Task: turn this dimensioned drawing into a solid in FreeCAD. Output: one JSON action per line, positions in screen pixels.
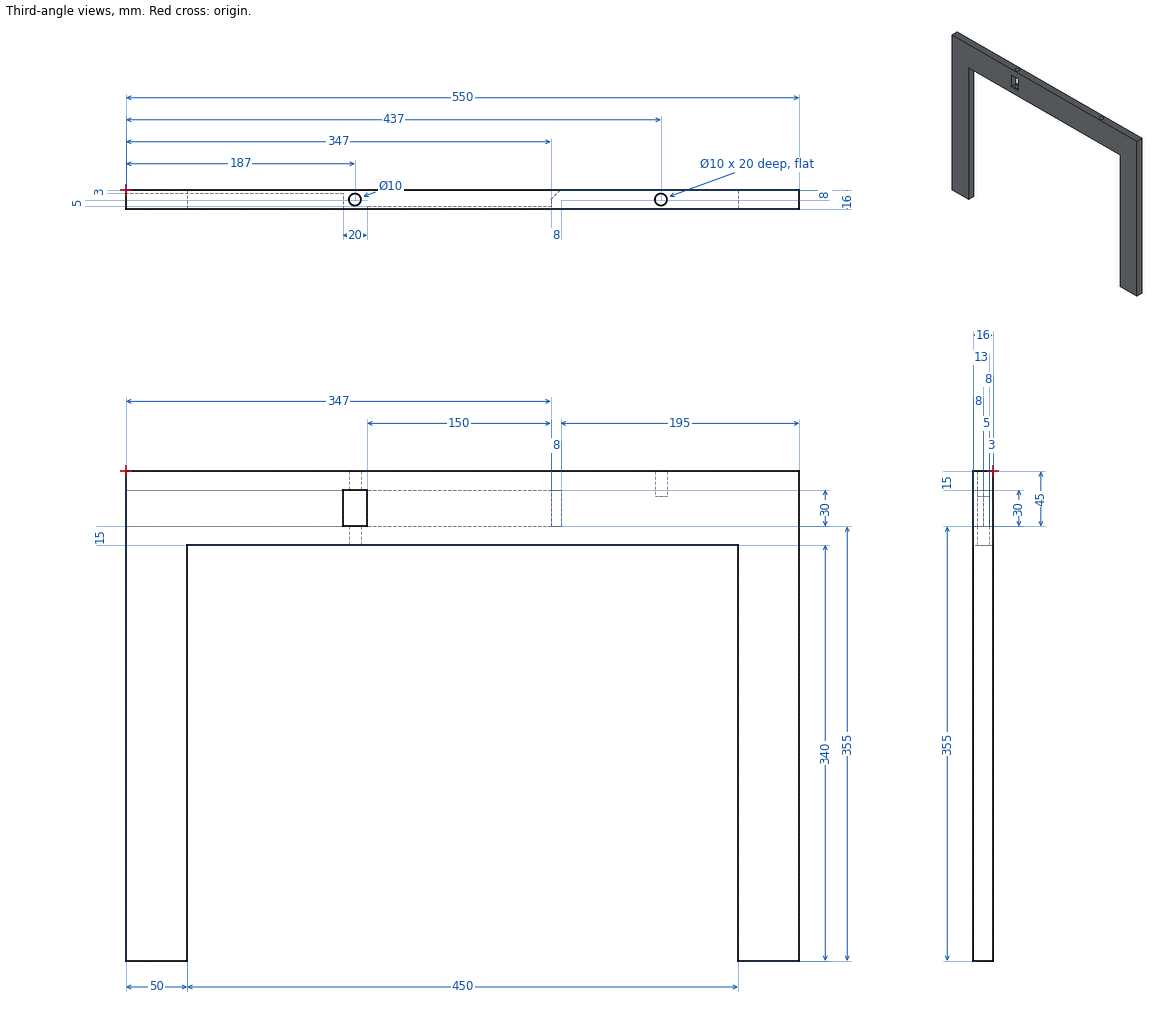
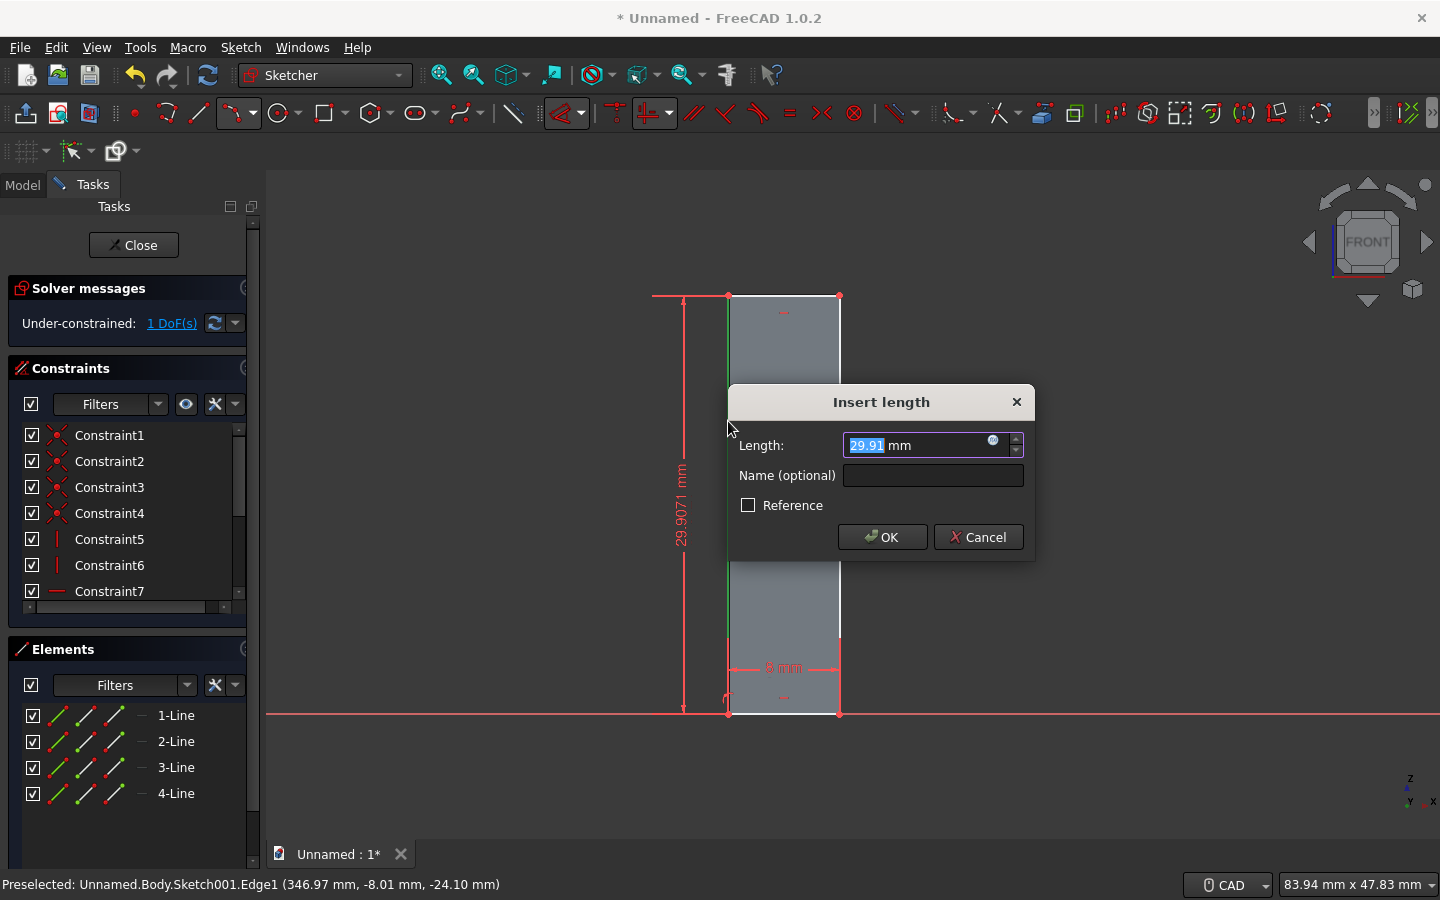
{"action": "type", "text": "30"}
{"action": "key", "text": "Return"}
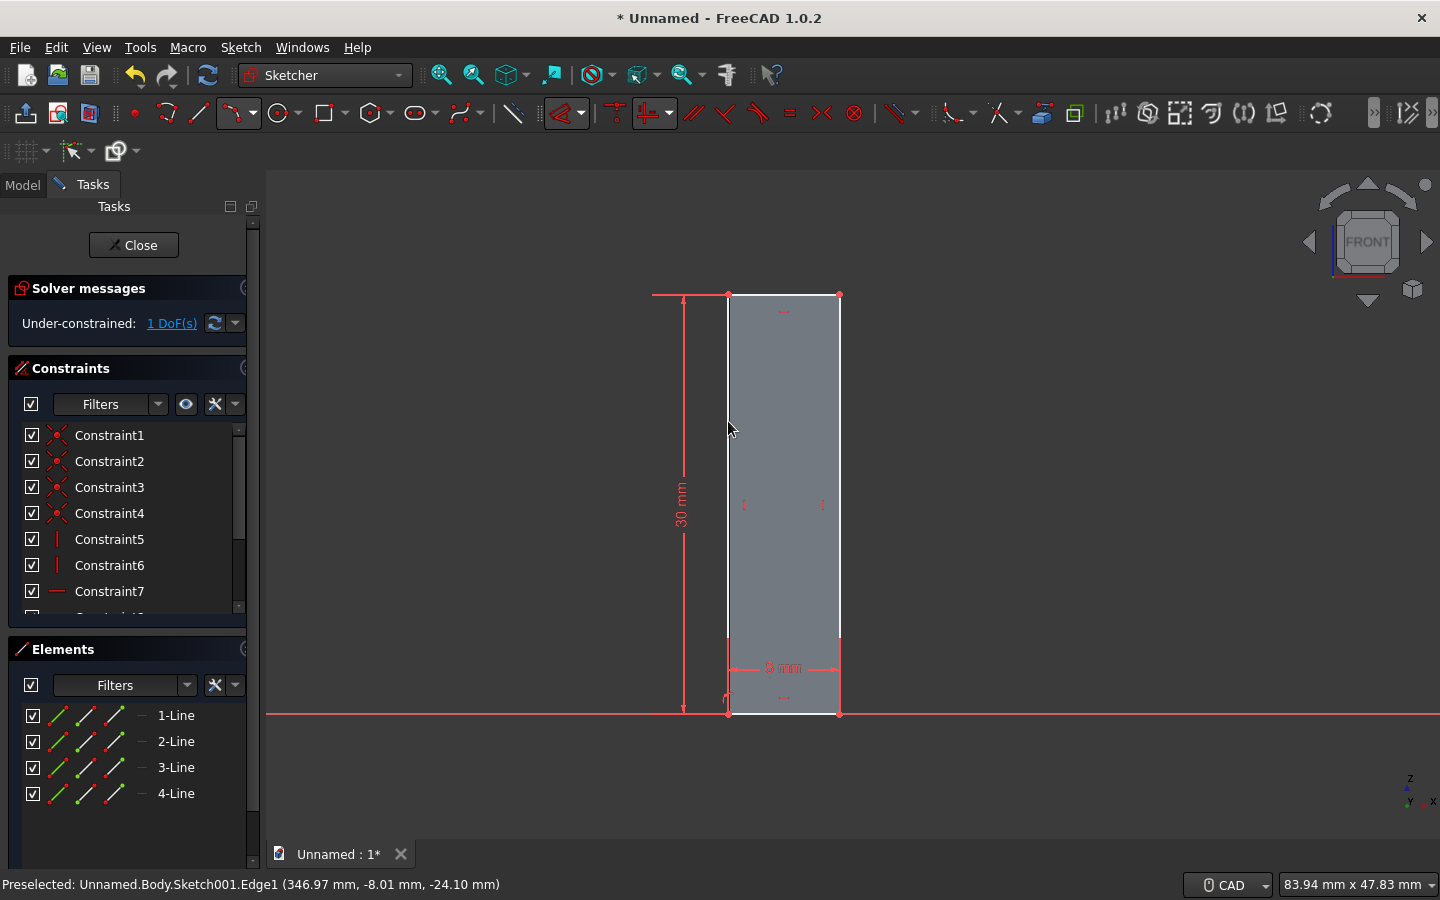
{"action": "left_click", "coordinate": [728, 295]}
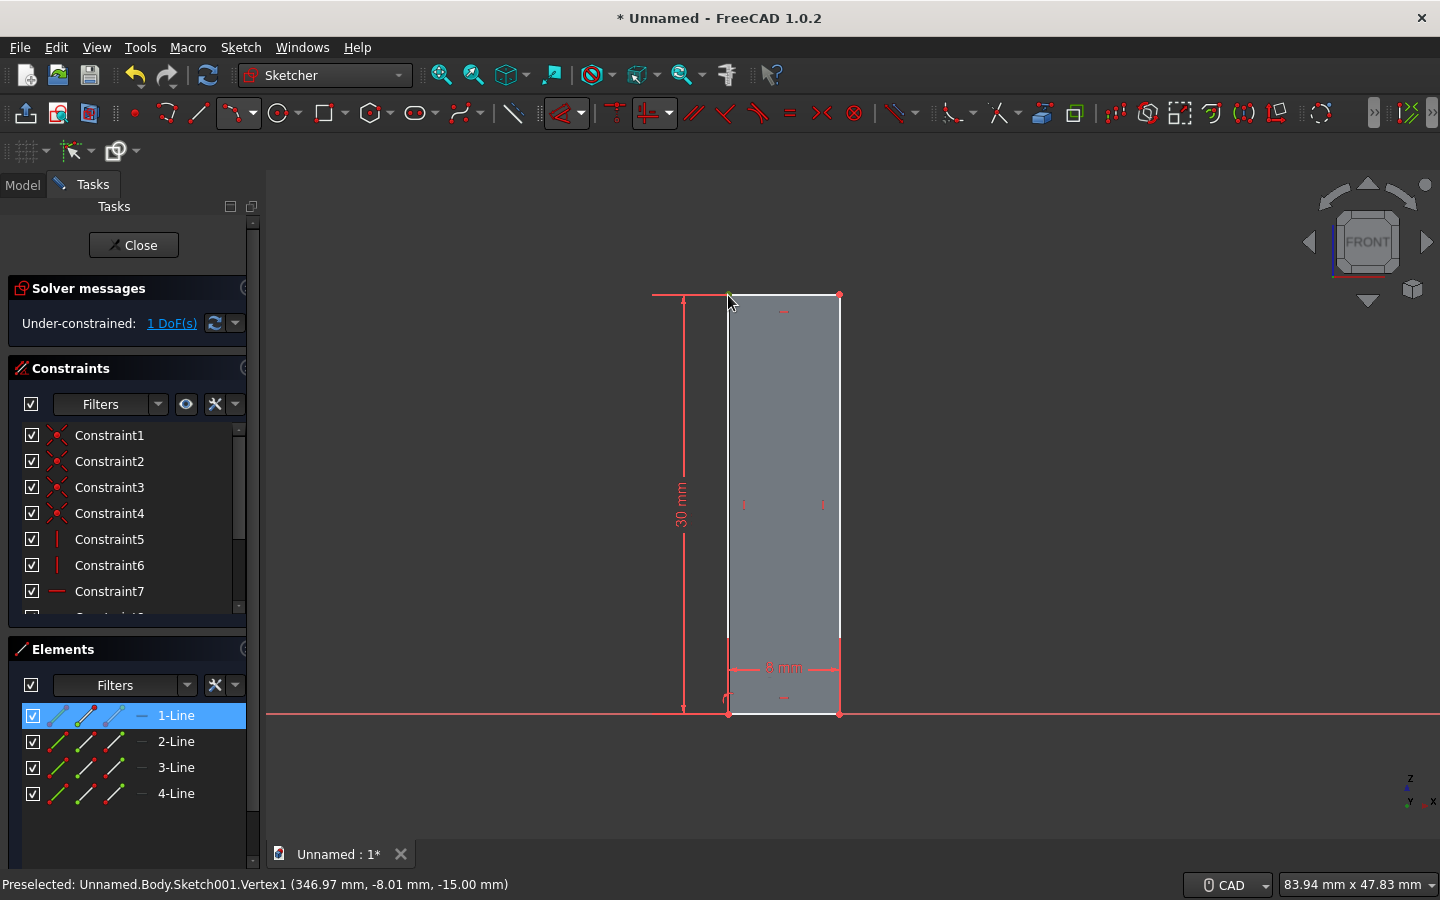
{"action": "left_click", "coordinate": [584, 114]}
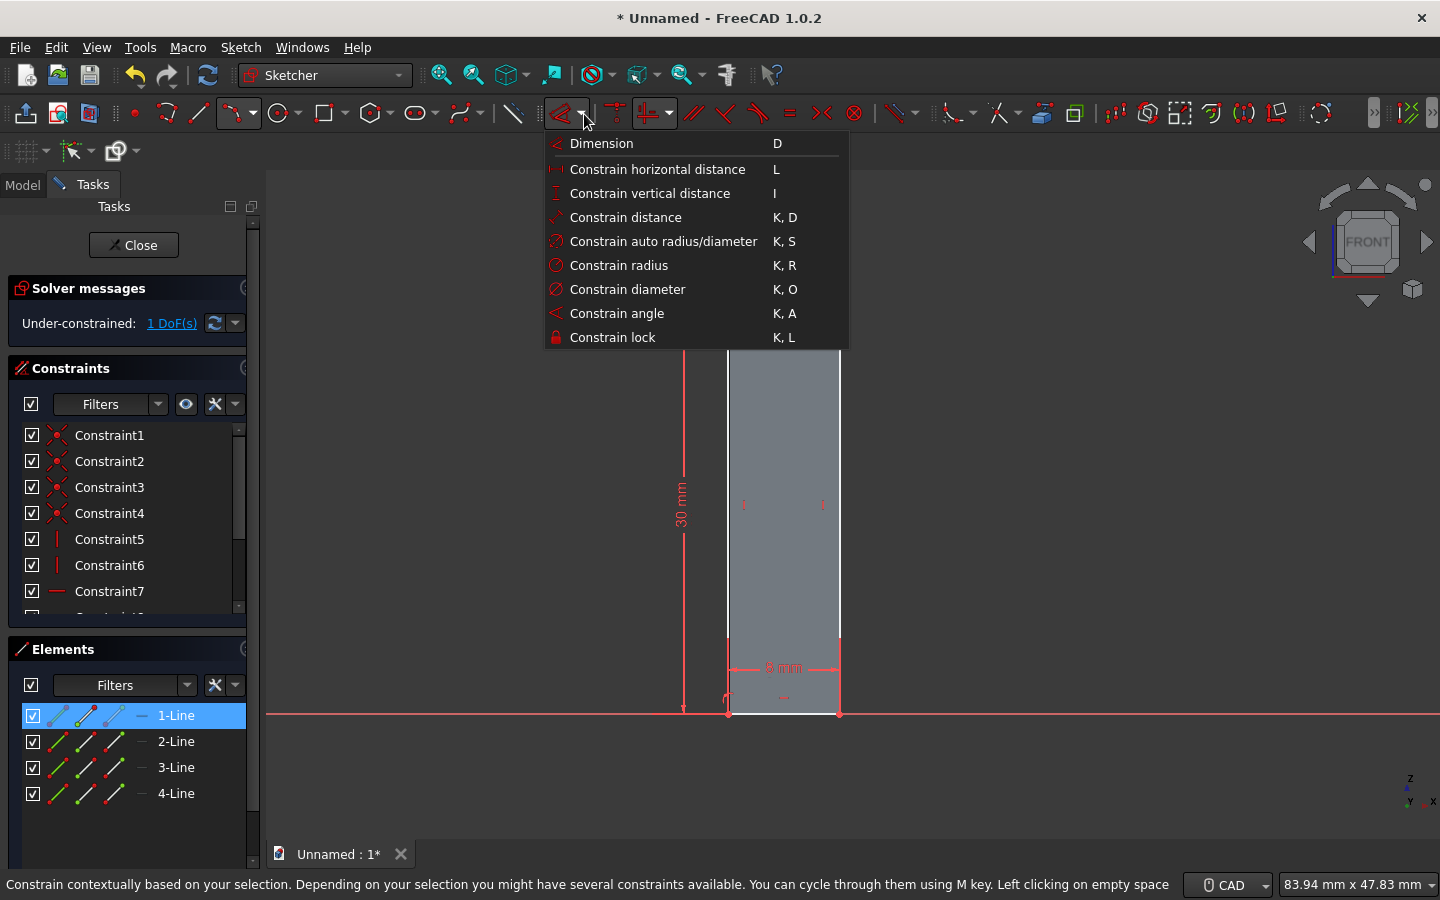
{"action": "left_click", "coordinate": [697, 169]}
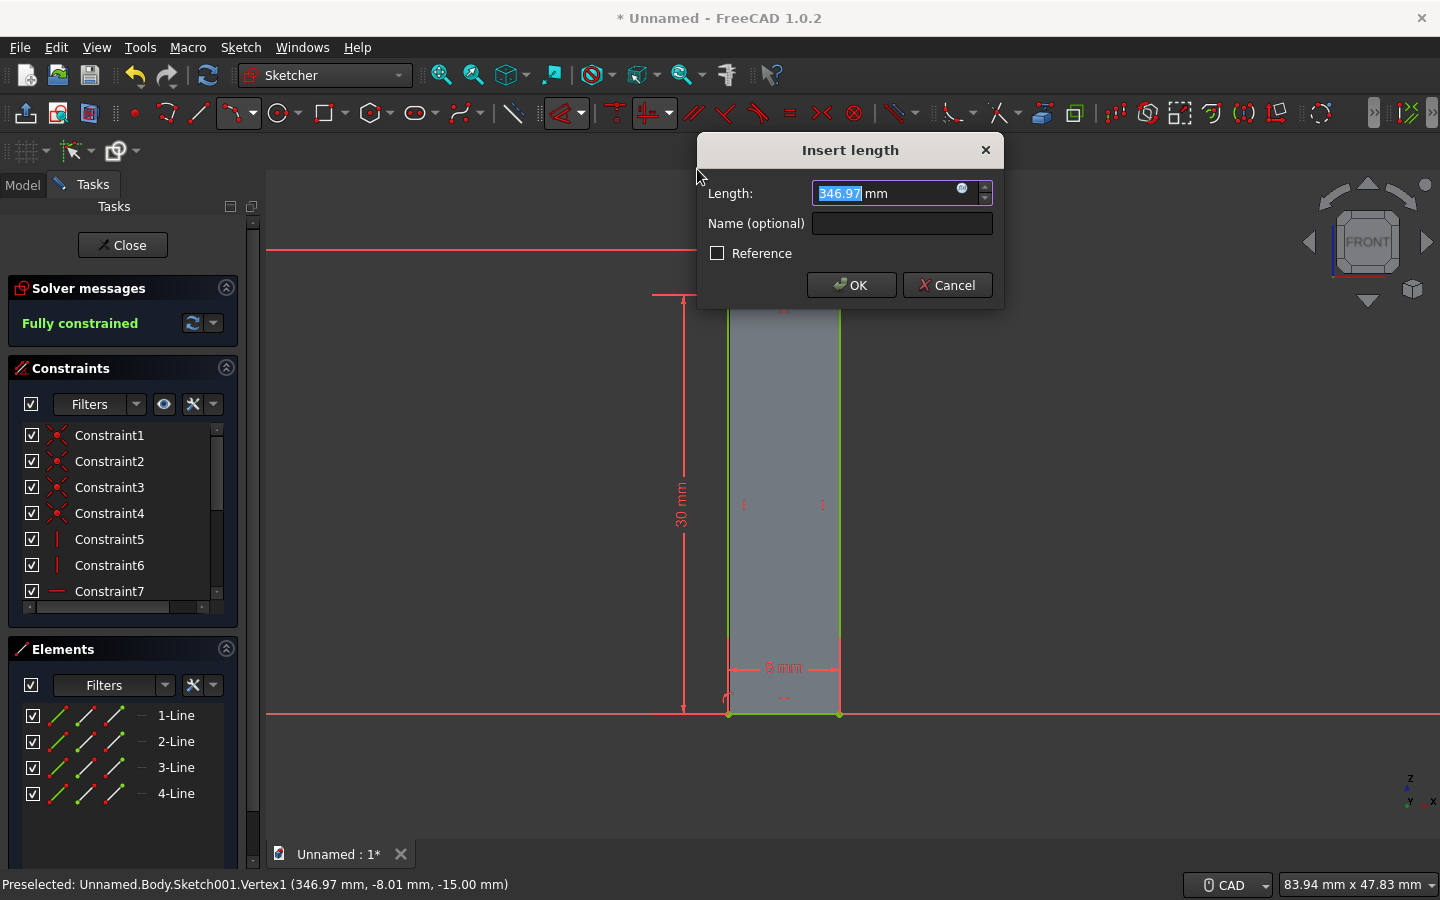
{"action": "type", "text": "347"}
{"action": "key", "text": "Return"}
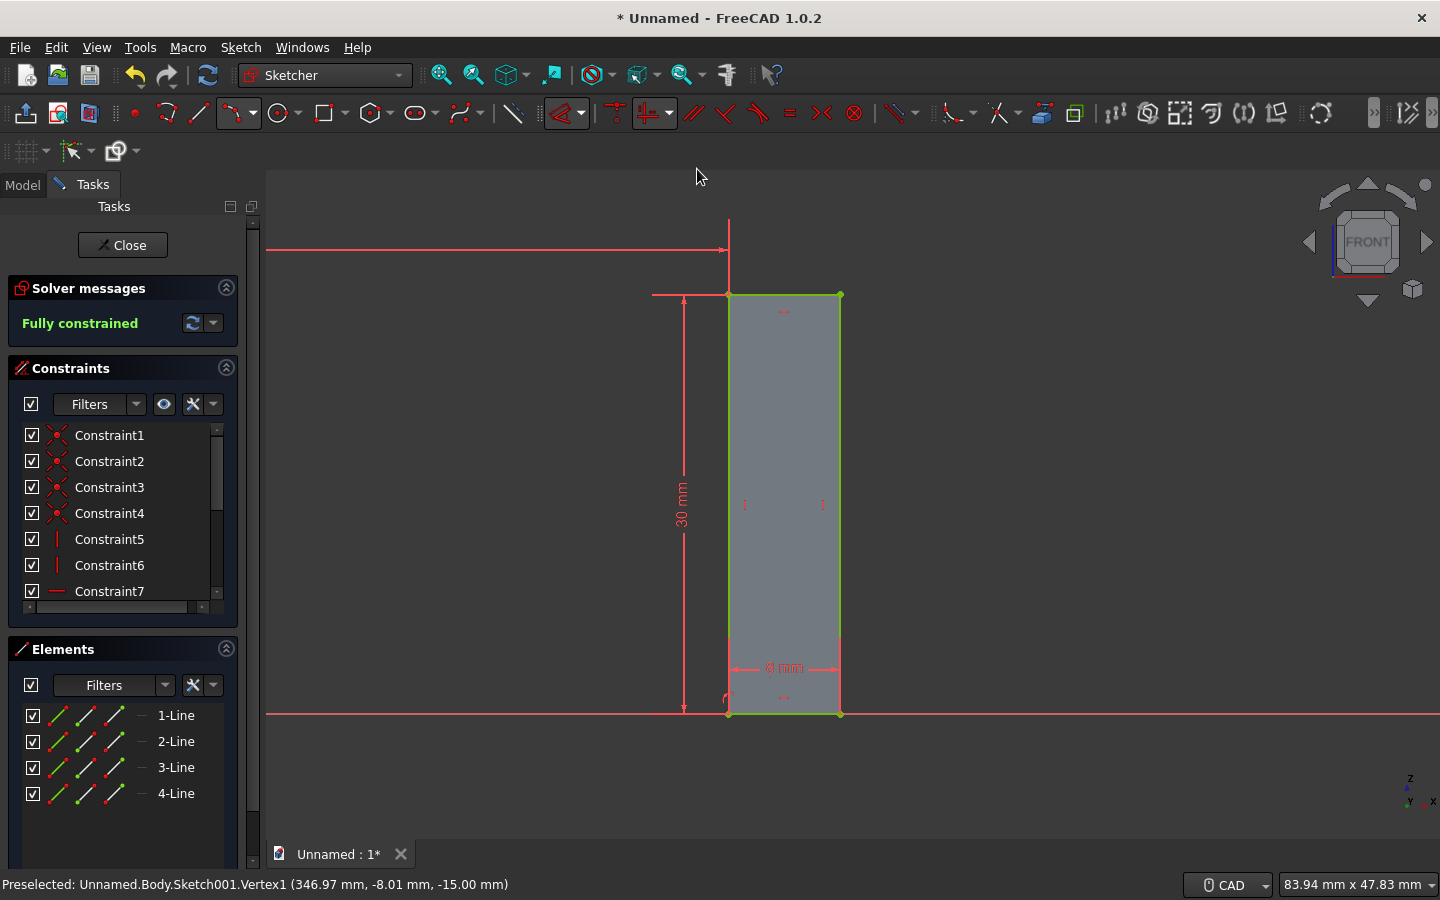
{"action": "left_click", "coordinate": [123, 245]}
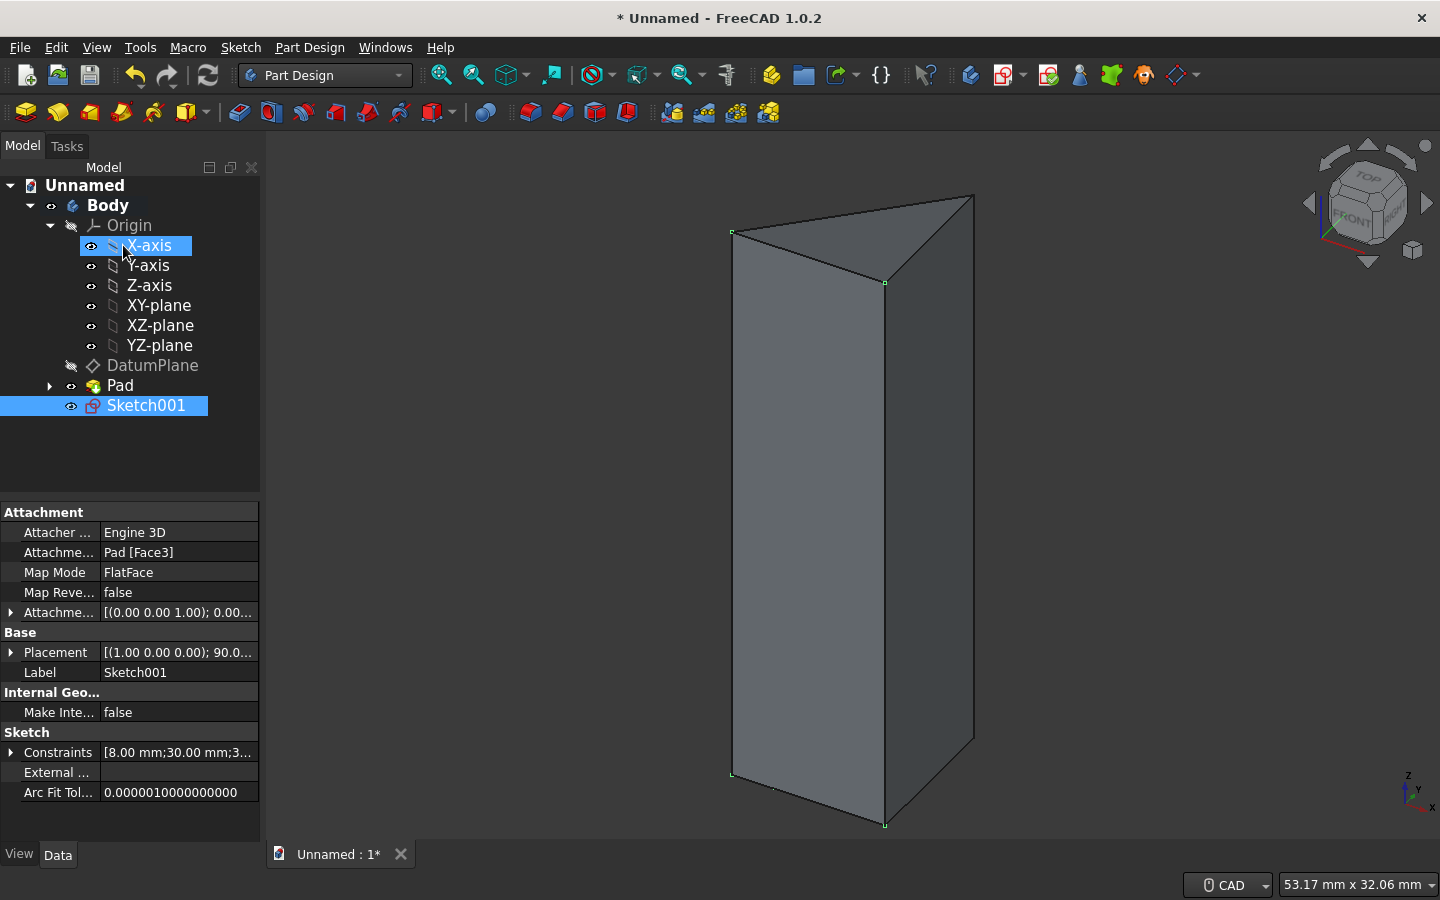
{"action": "left_click", "coordinate": [26, 112]}